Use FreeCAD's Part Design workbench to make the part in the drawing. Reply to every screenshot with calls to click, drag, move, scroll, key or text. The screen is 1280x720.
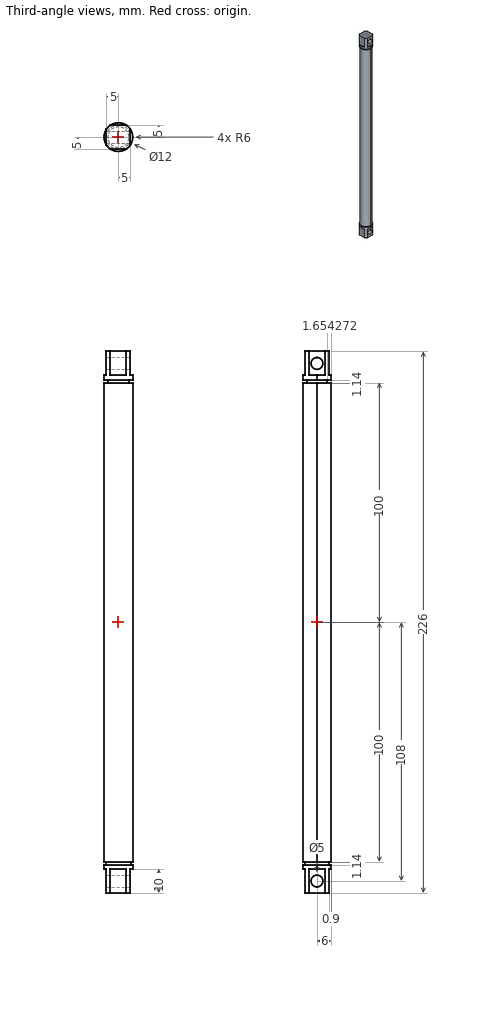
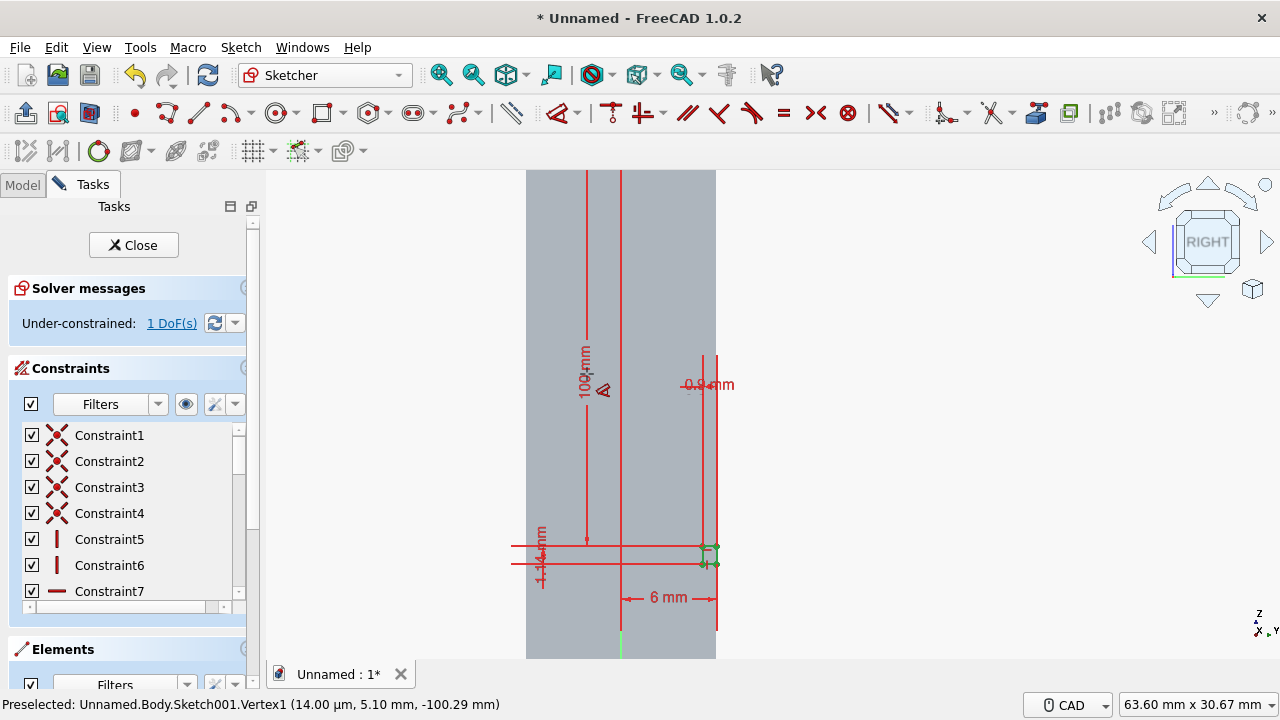
scroll(708, 560, down, 12)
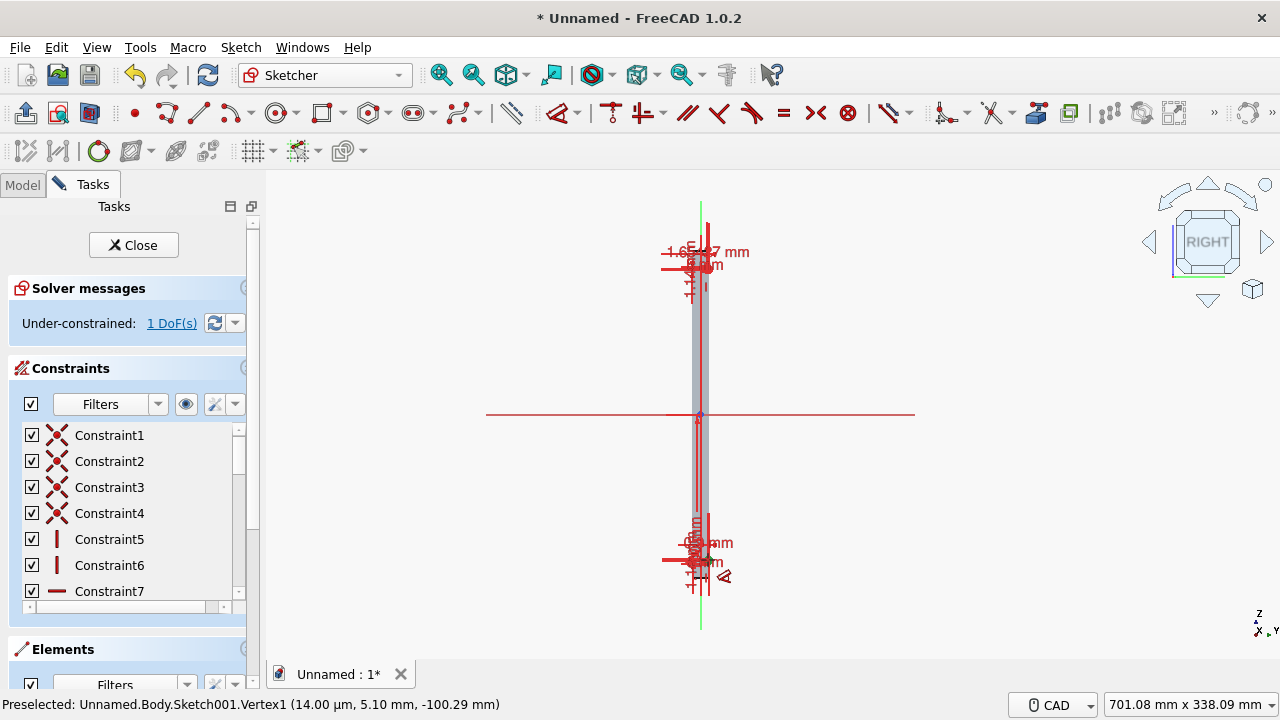
scroll(707, 270, up, 11)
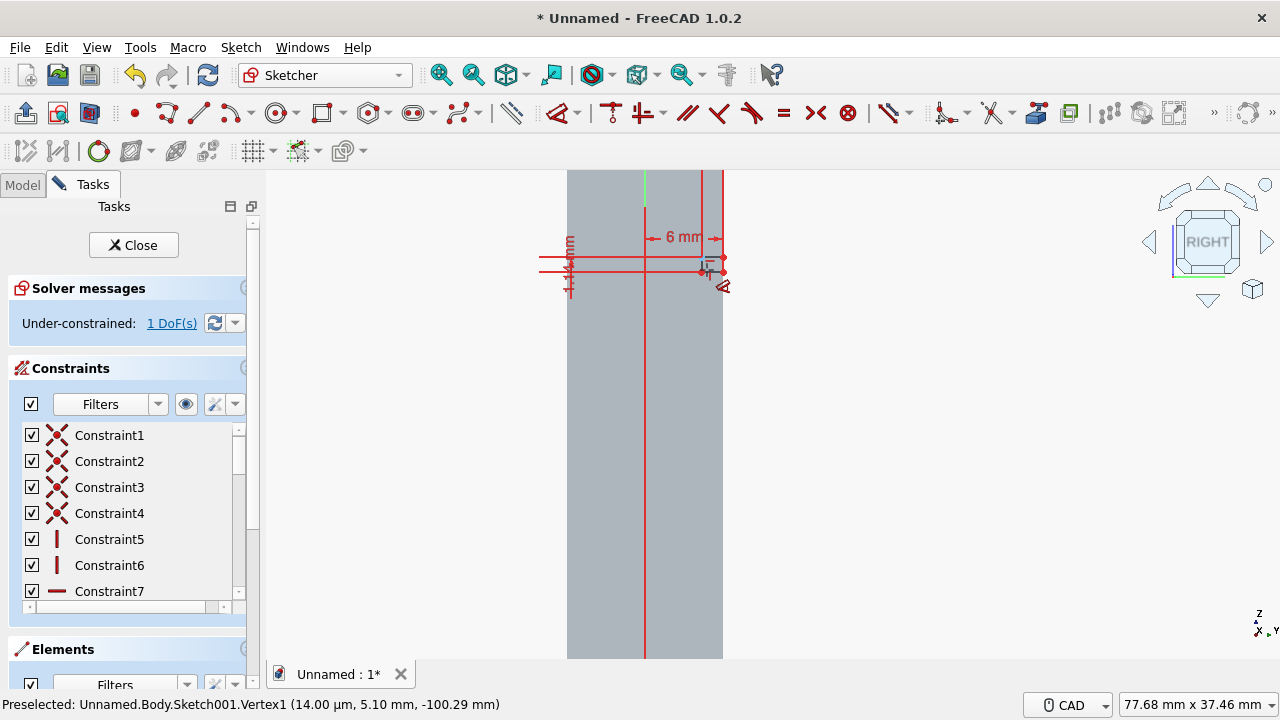
click(702, 272)
click(611, 452)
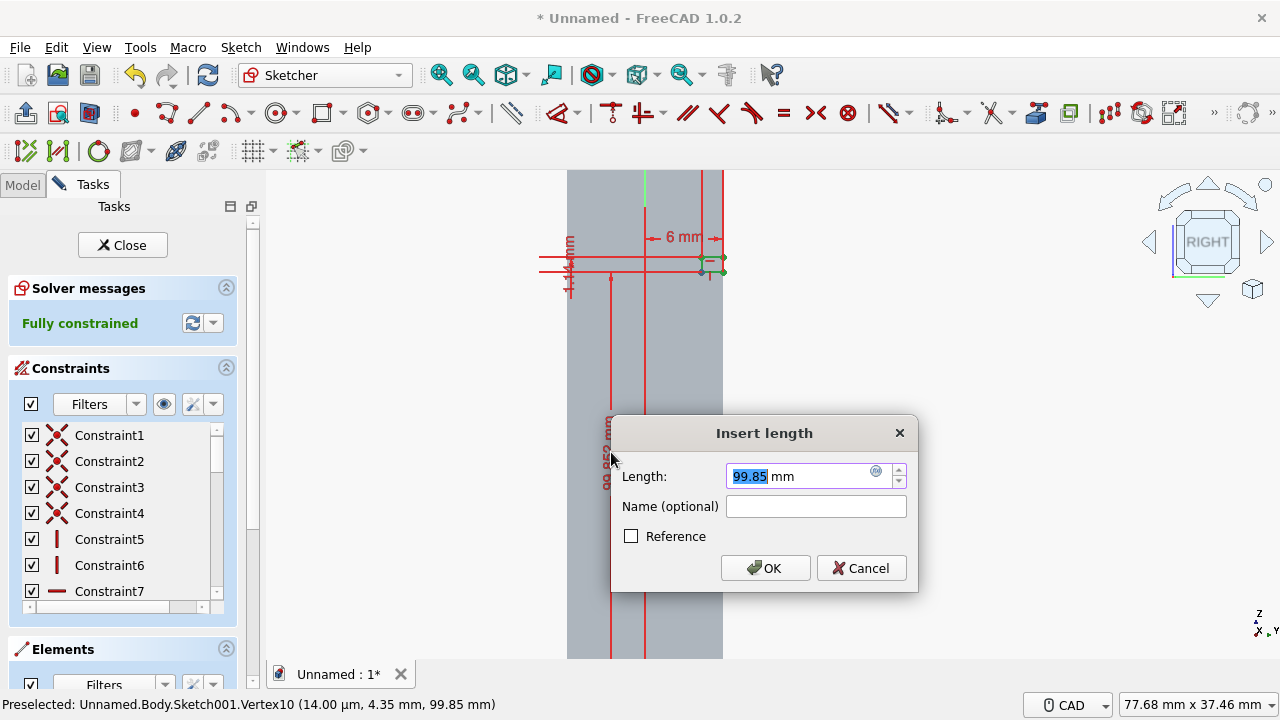
text(100)
key(Return)
key(Escape)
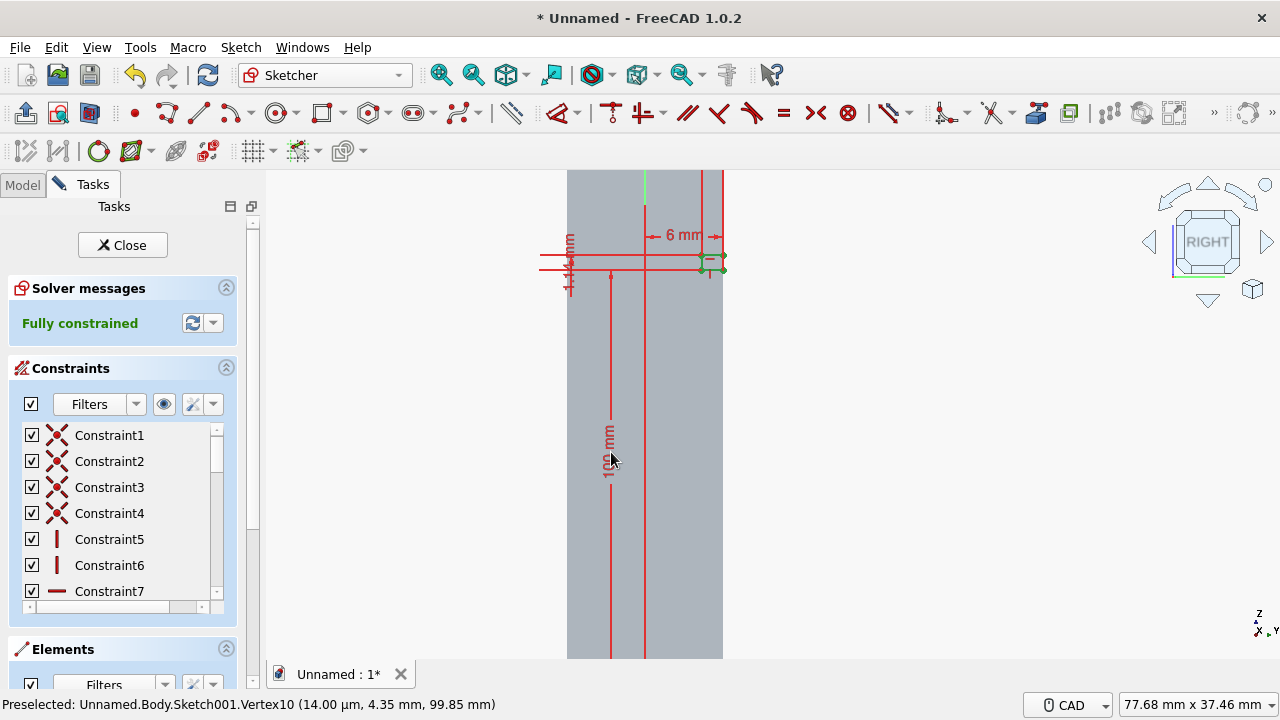
click(123, 245)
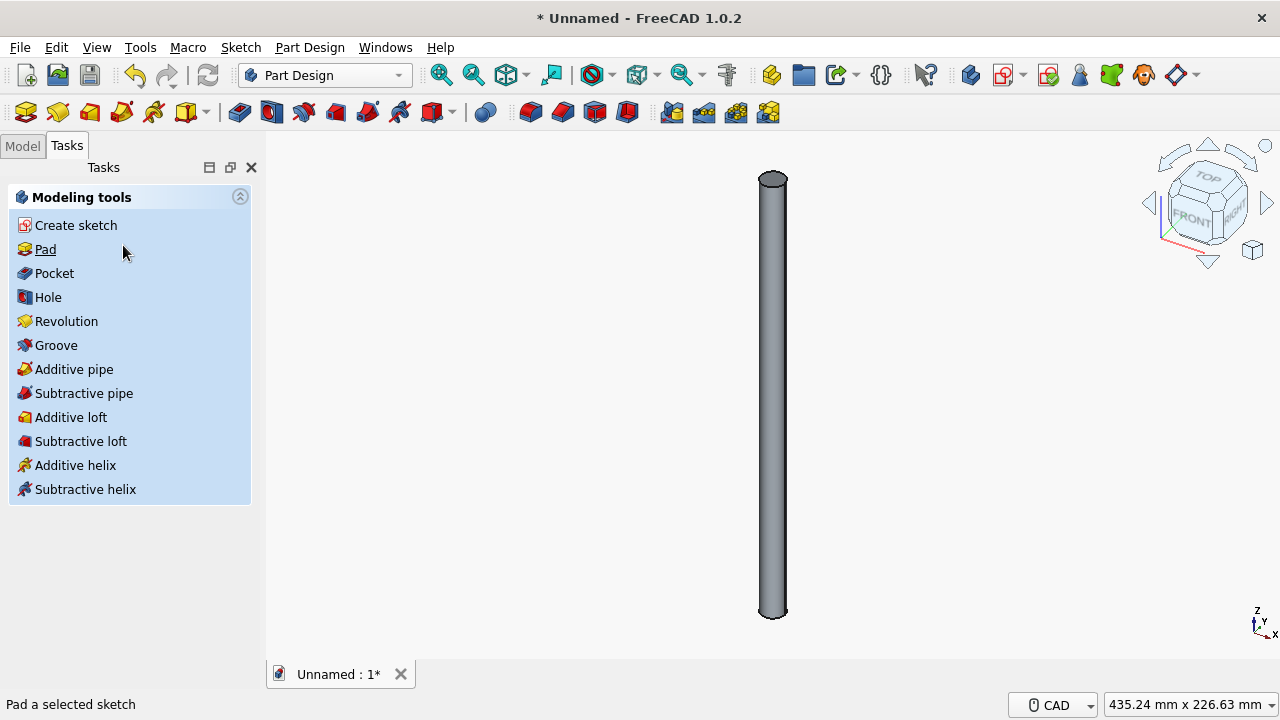
click(304, 112)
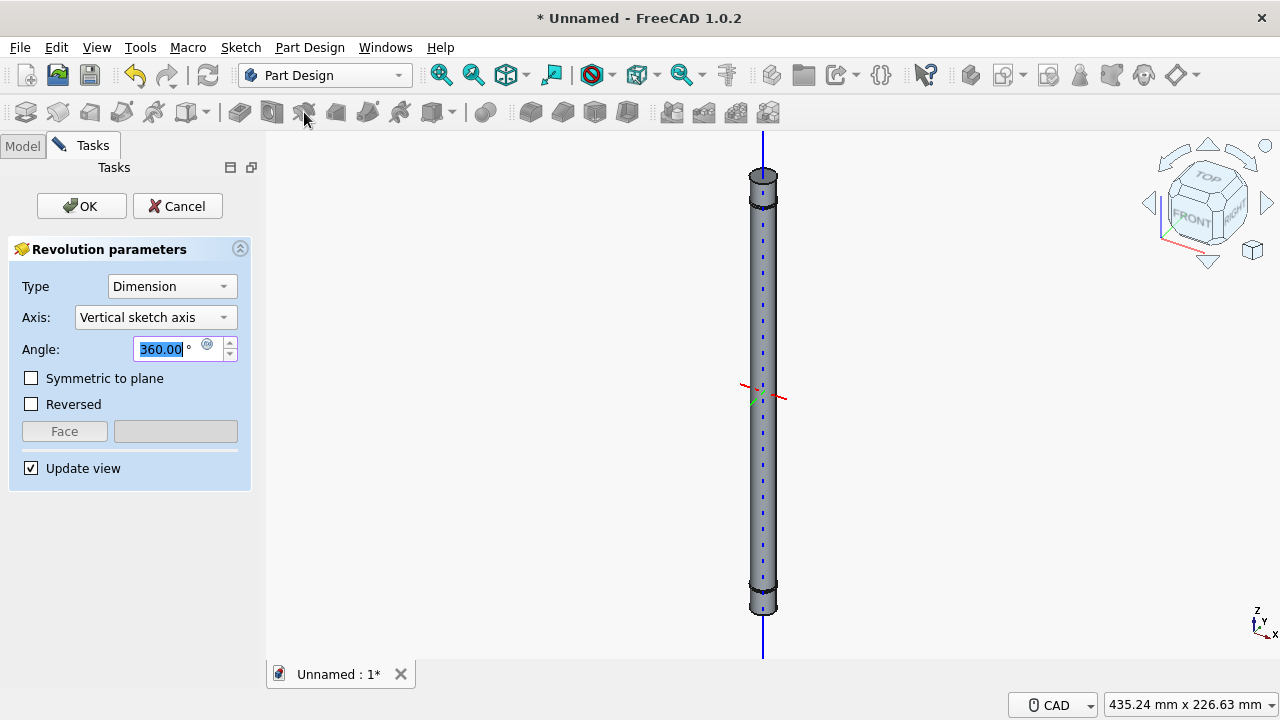
click(82, 206)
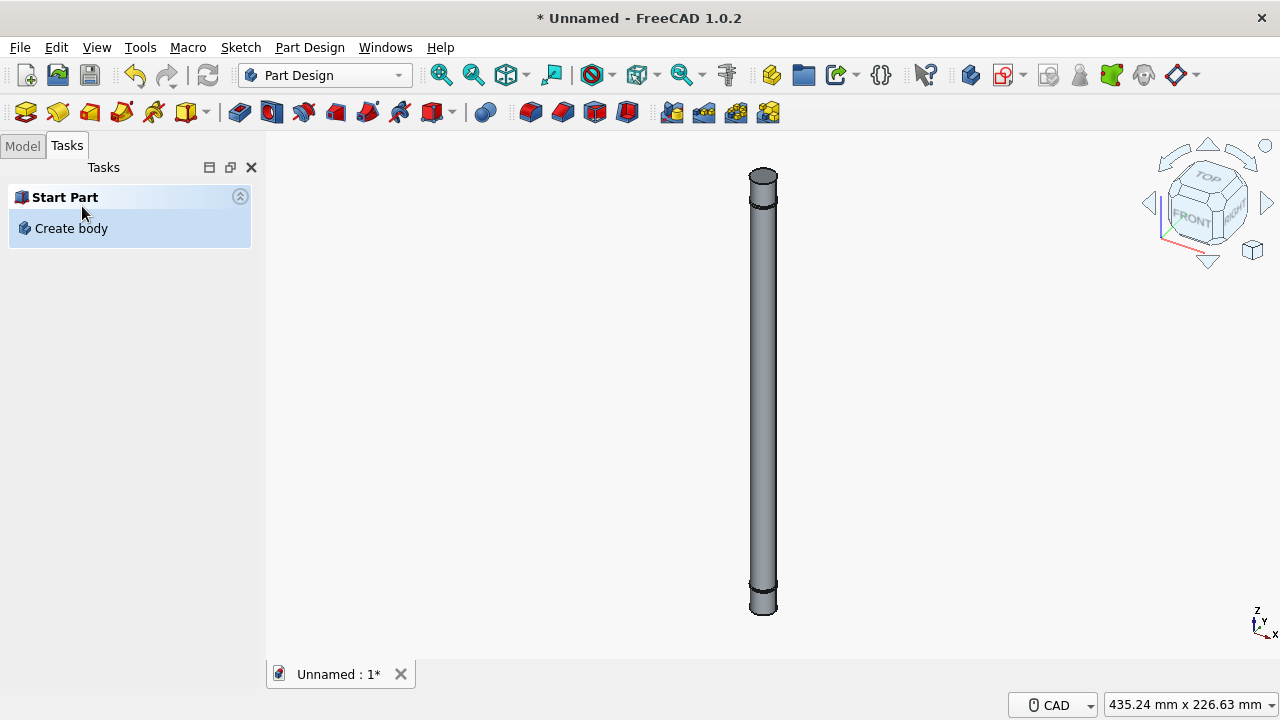
click(23, 145)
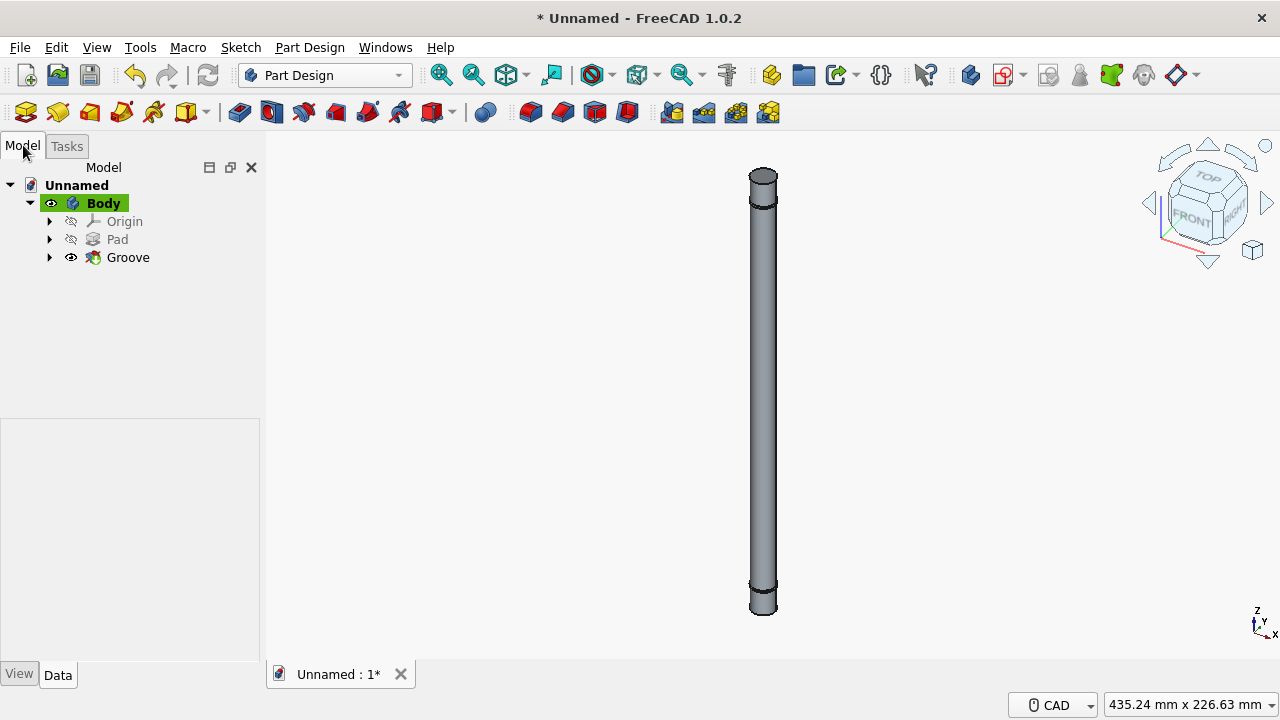
click(50, 221)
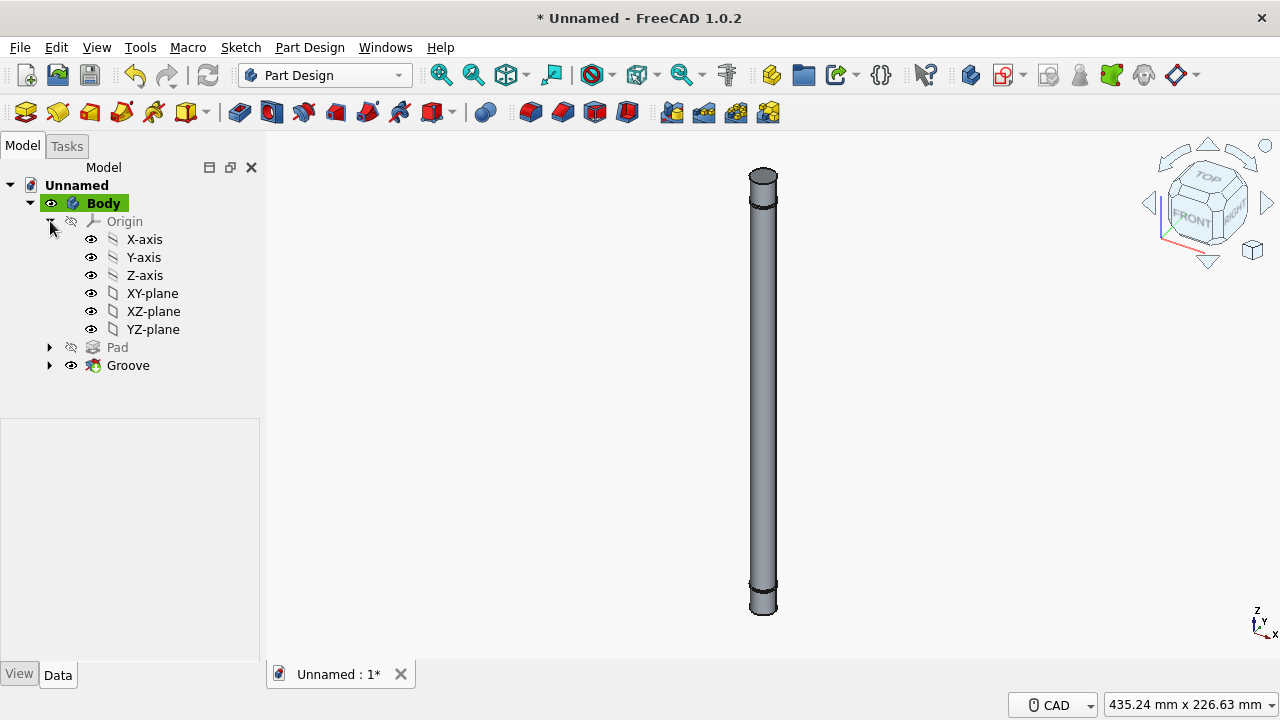
click(136, 293)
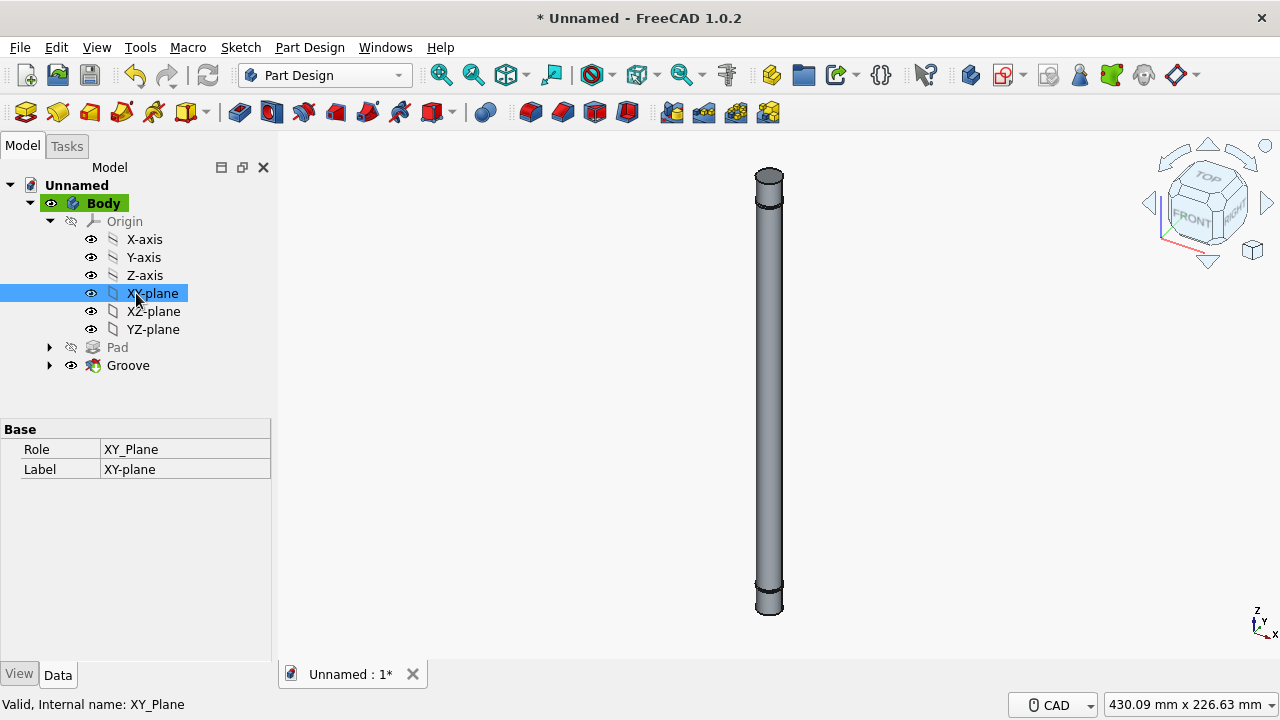
click(1176, 76)